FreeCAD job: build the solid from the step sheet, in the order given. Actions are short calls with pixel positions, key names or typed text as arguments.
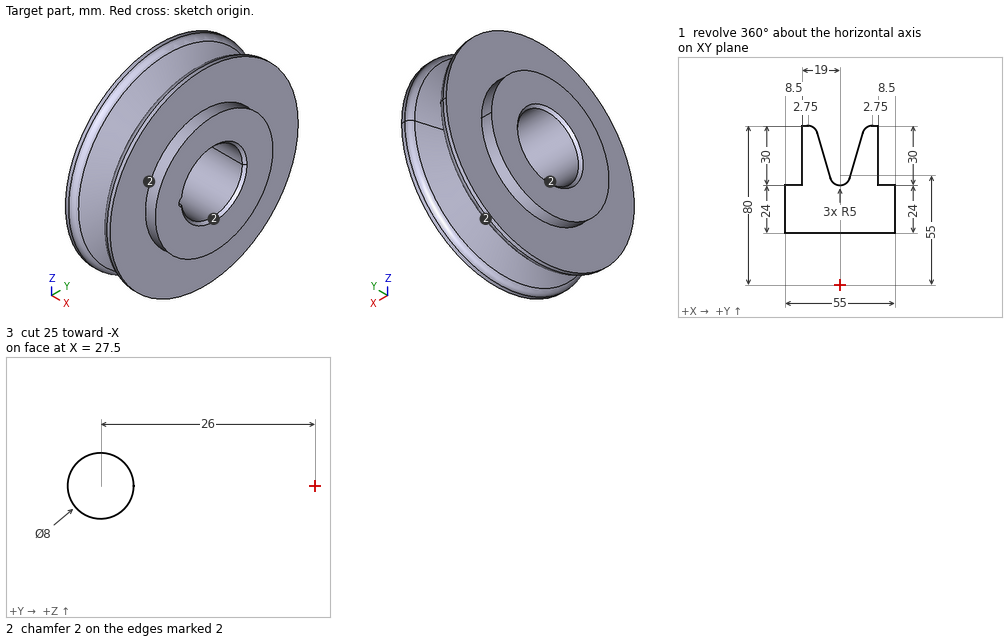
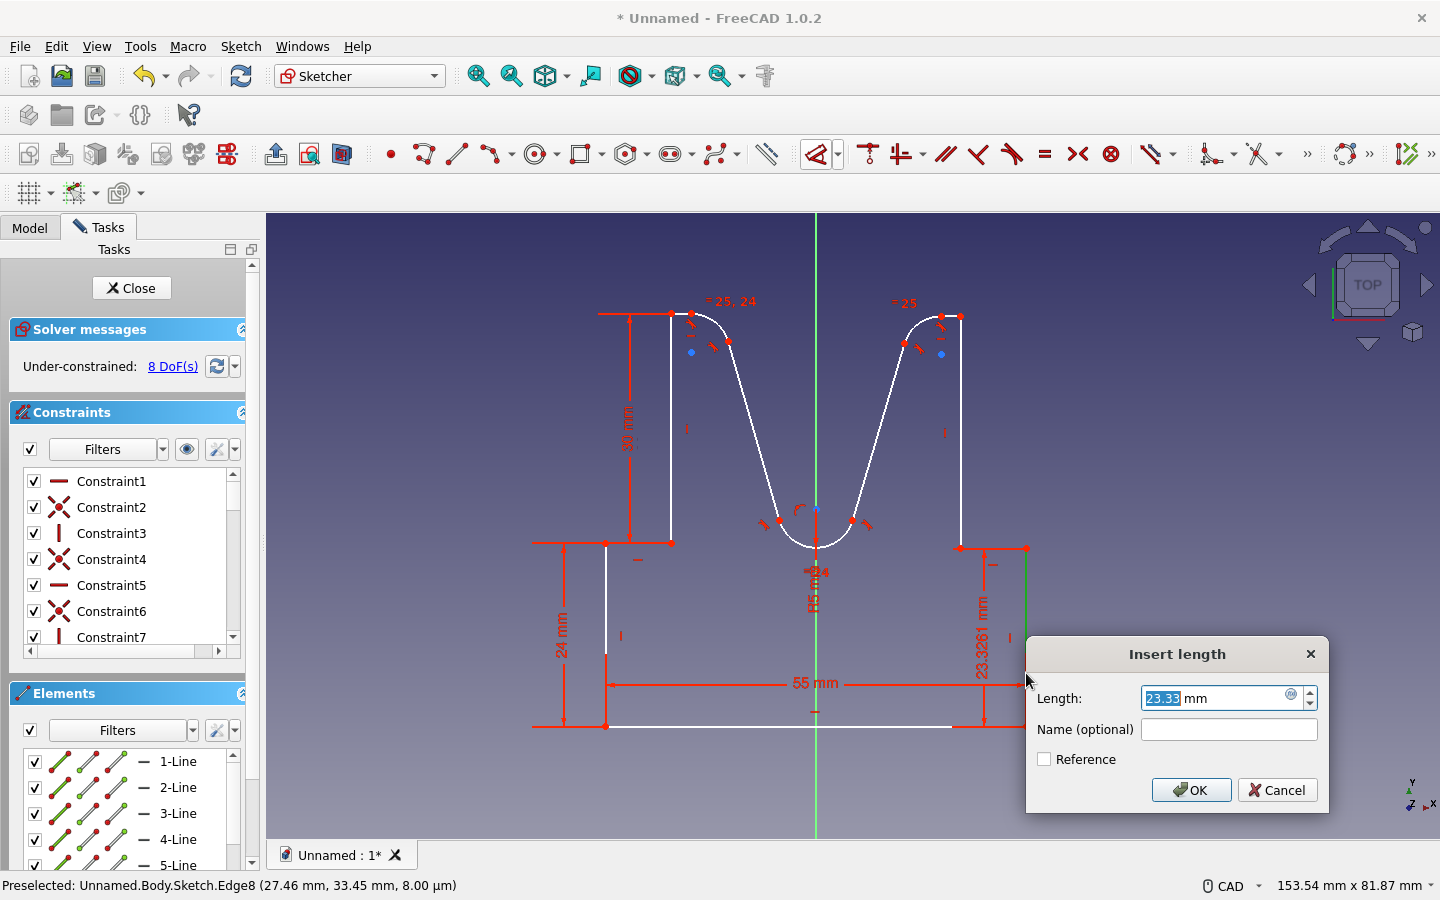
text(24)
key(Return)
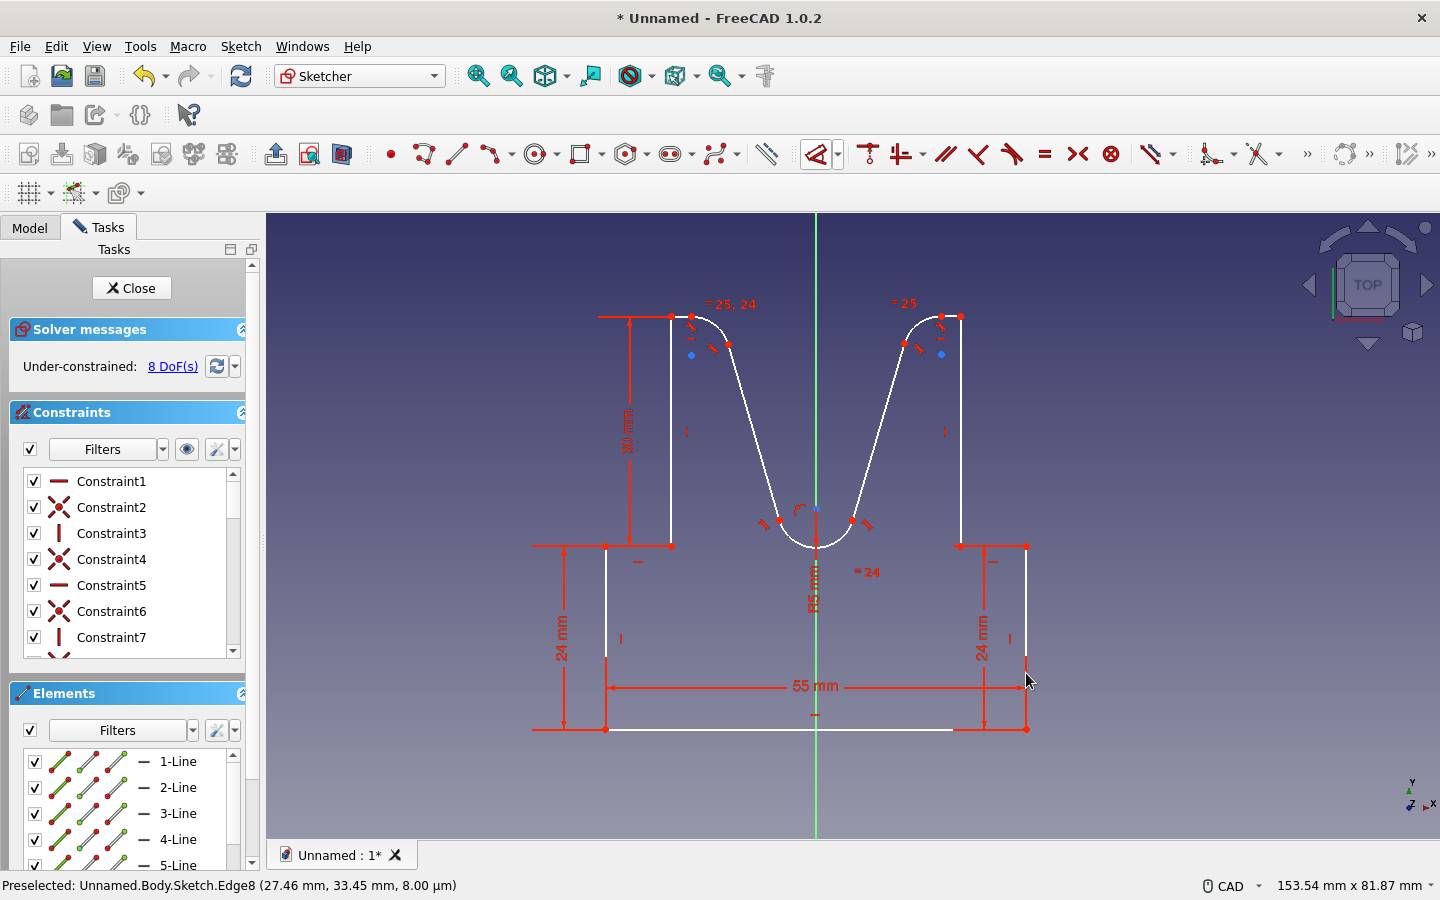
click(961, 477)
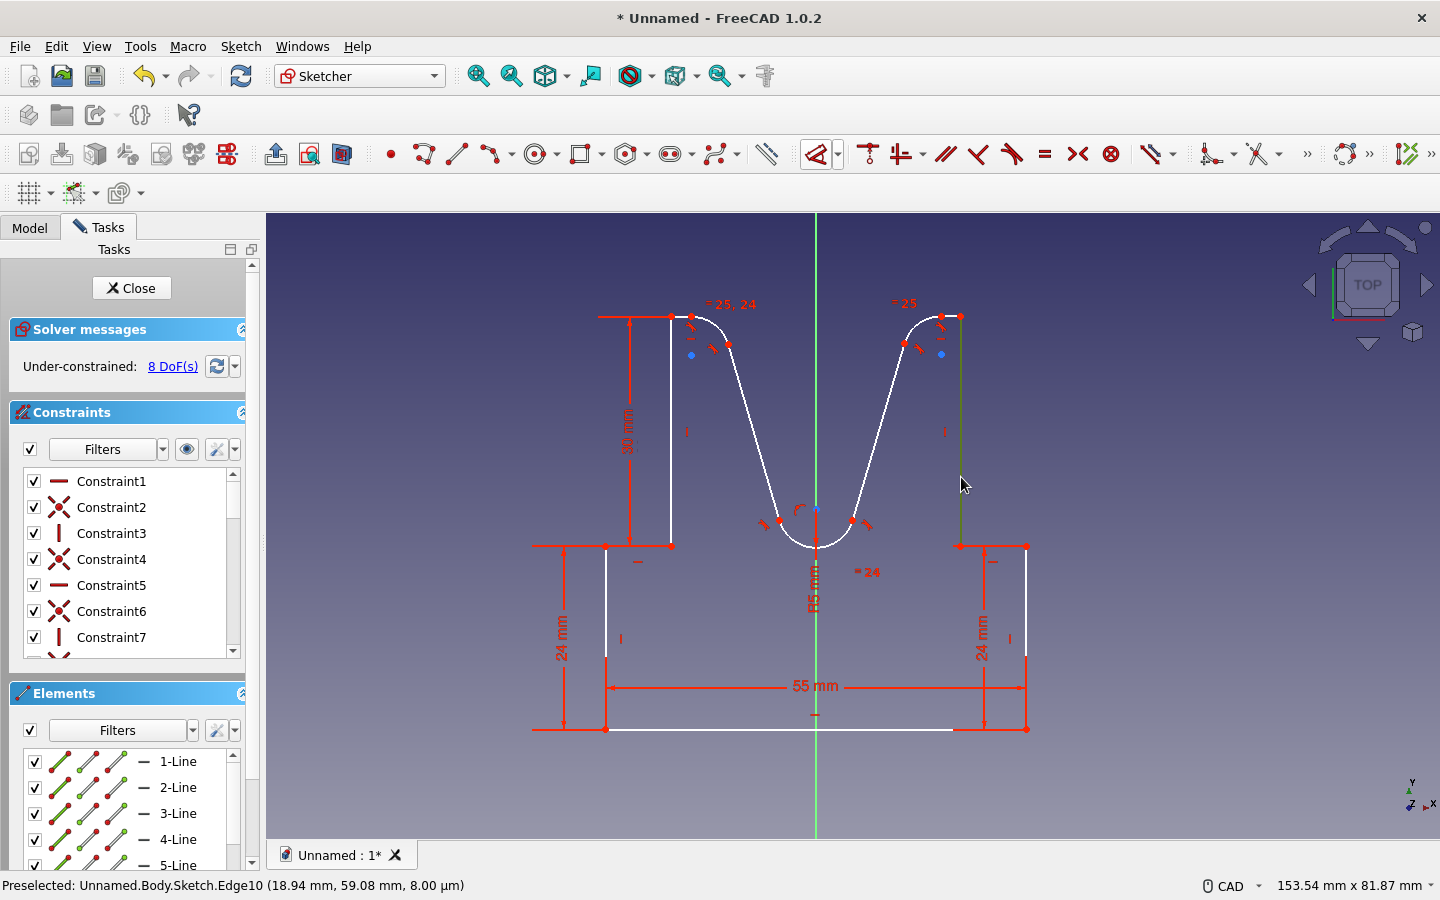
key(i)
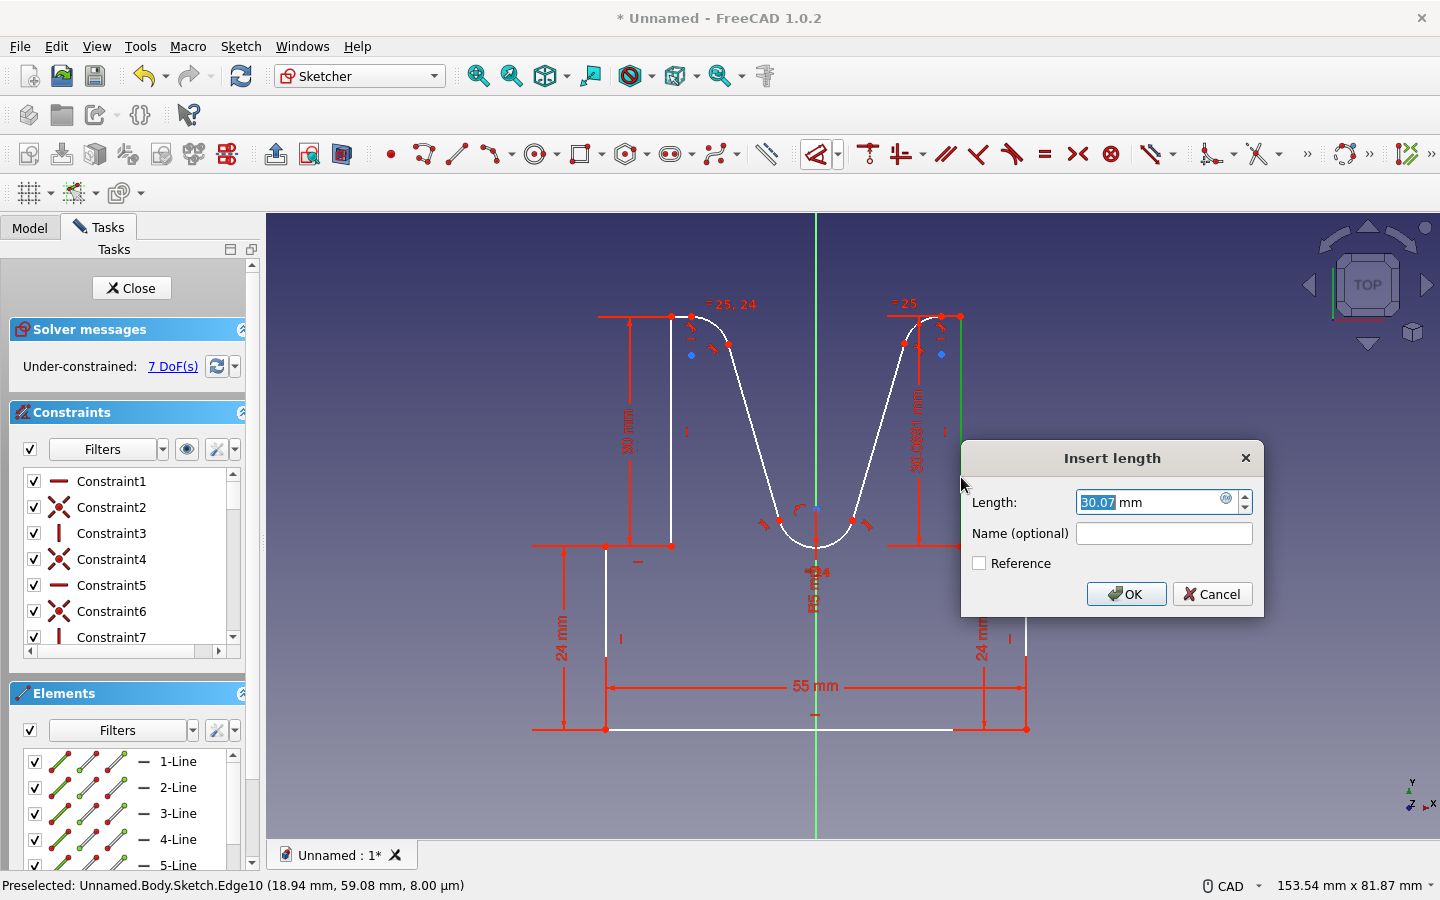
text(30)
key(Return)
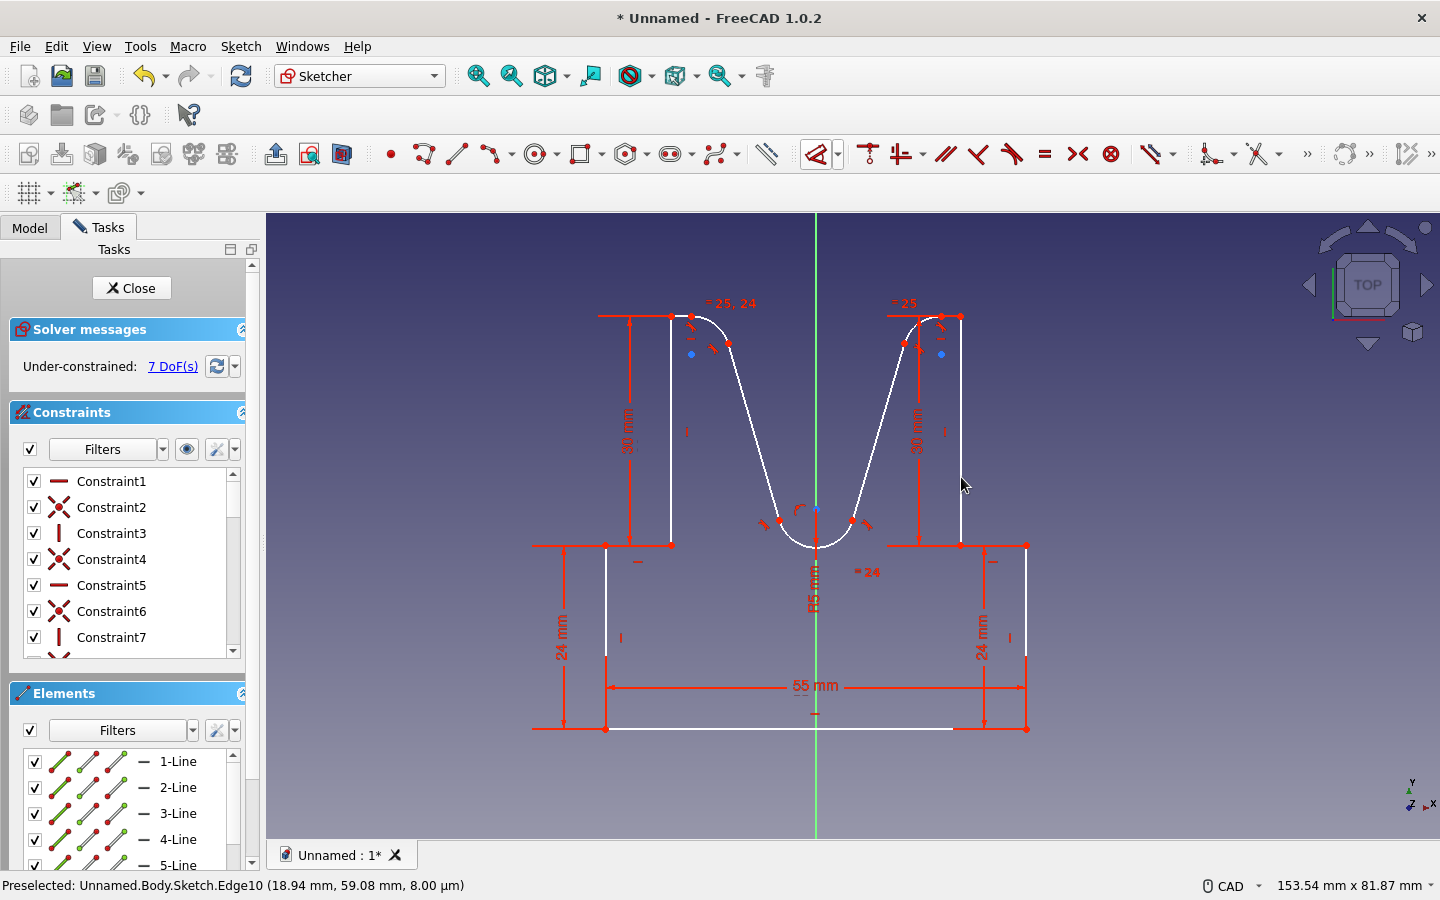
click(652, 546)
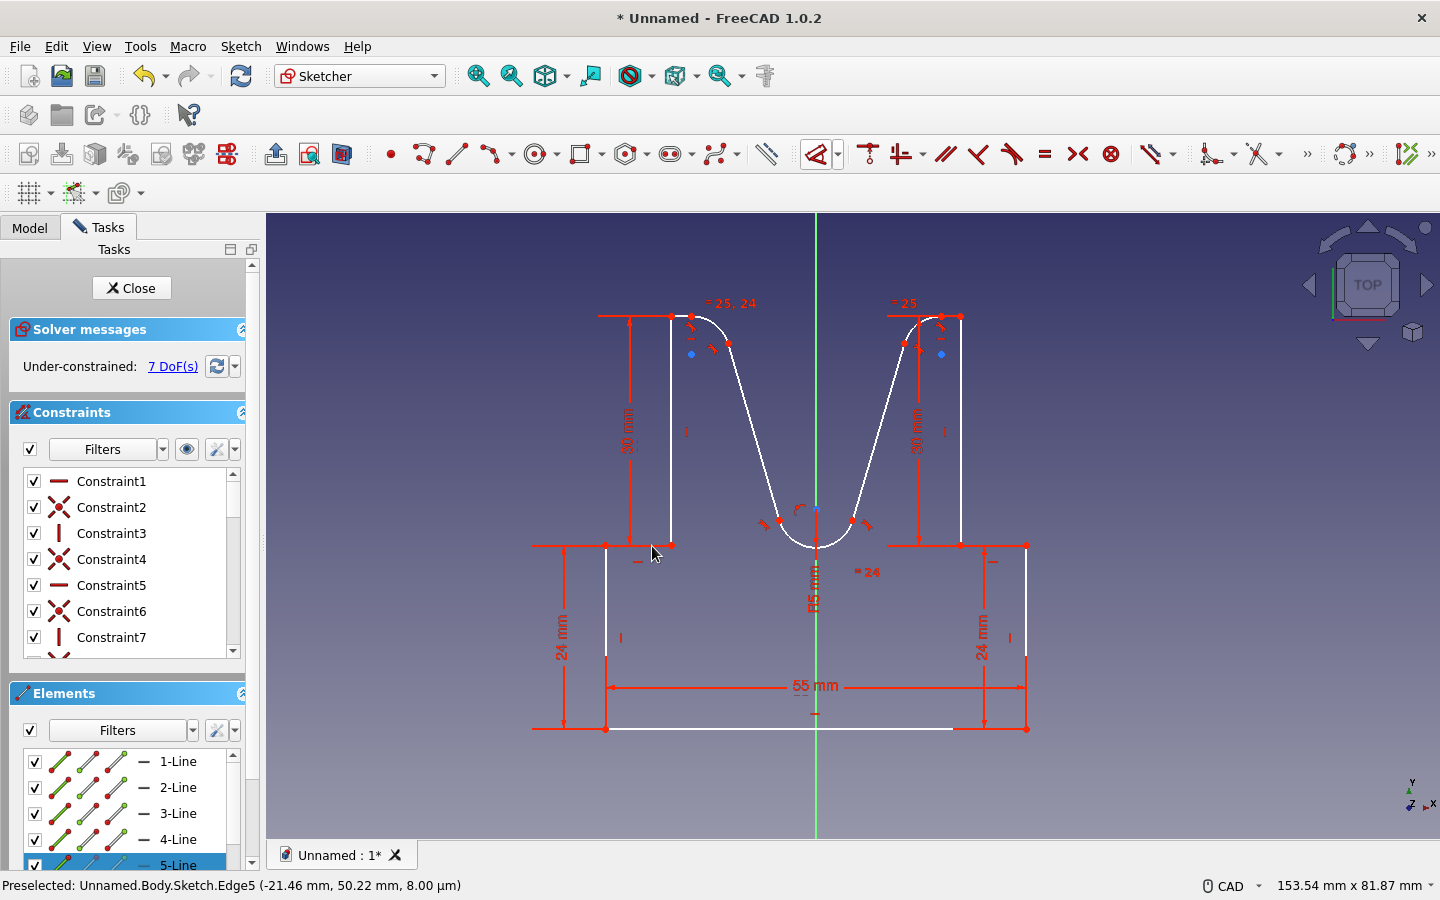
key(l)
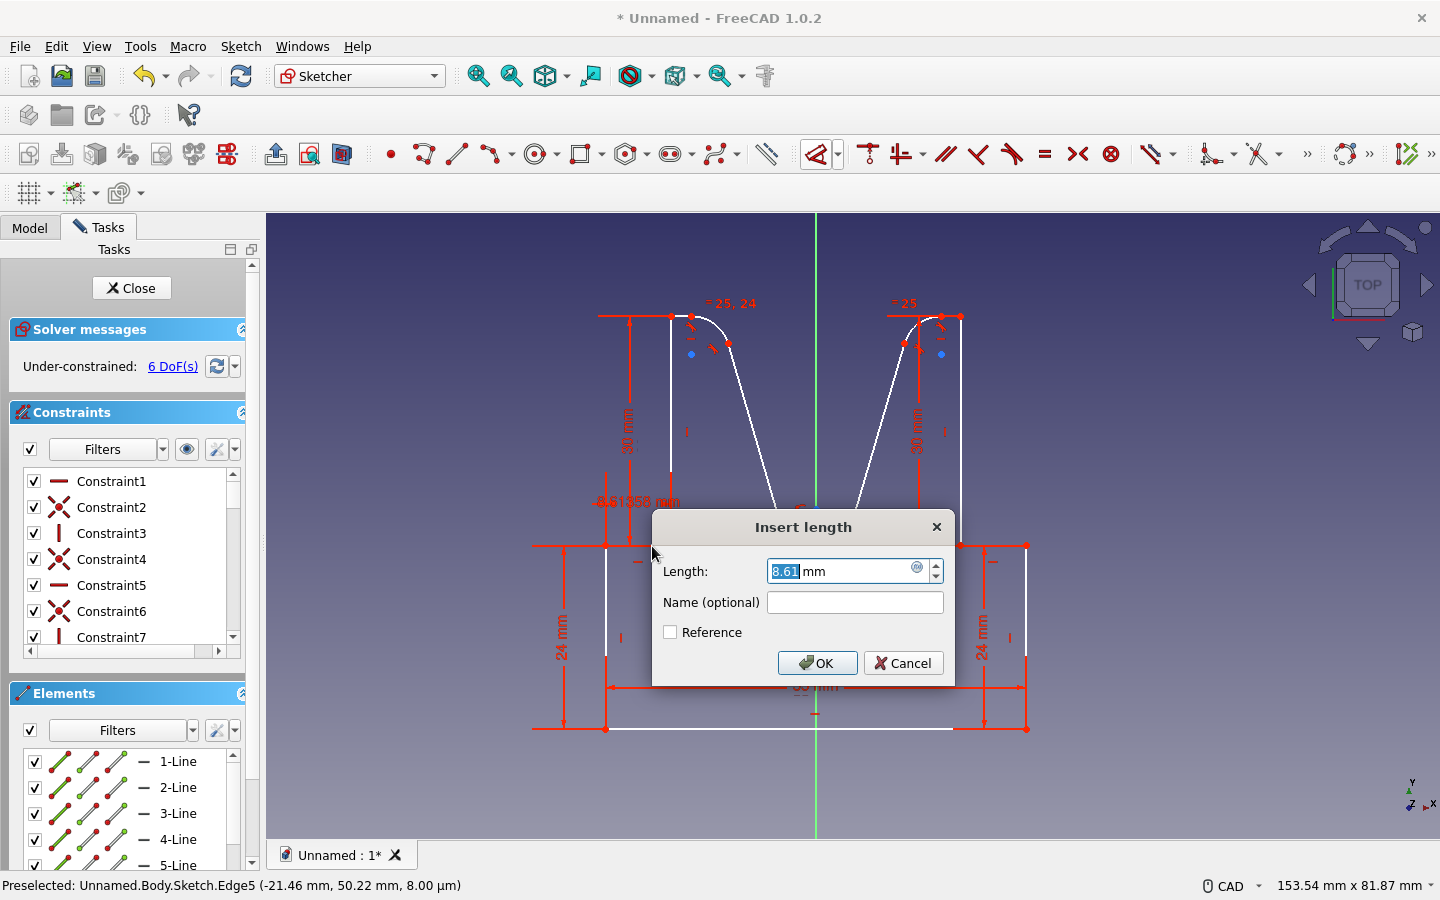
text(8.5)
key(Return)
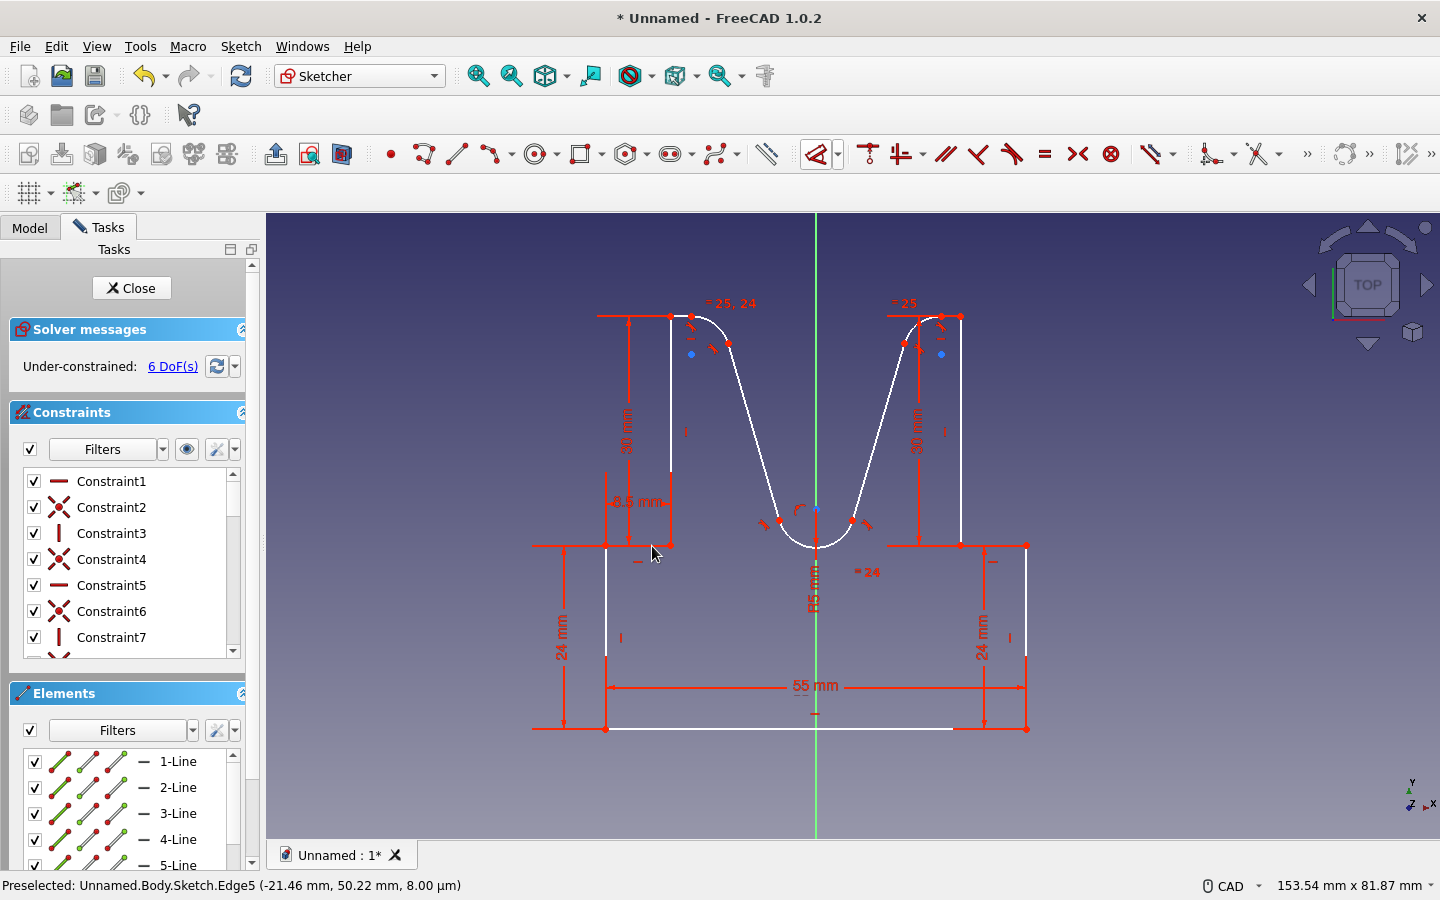
click(1007, 546)